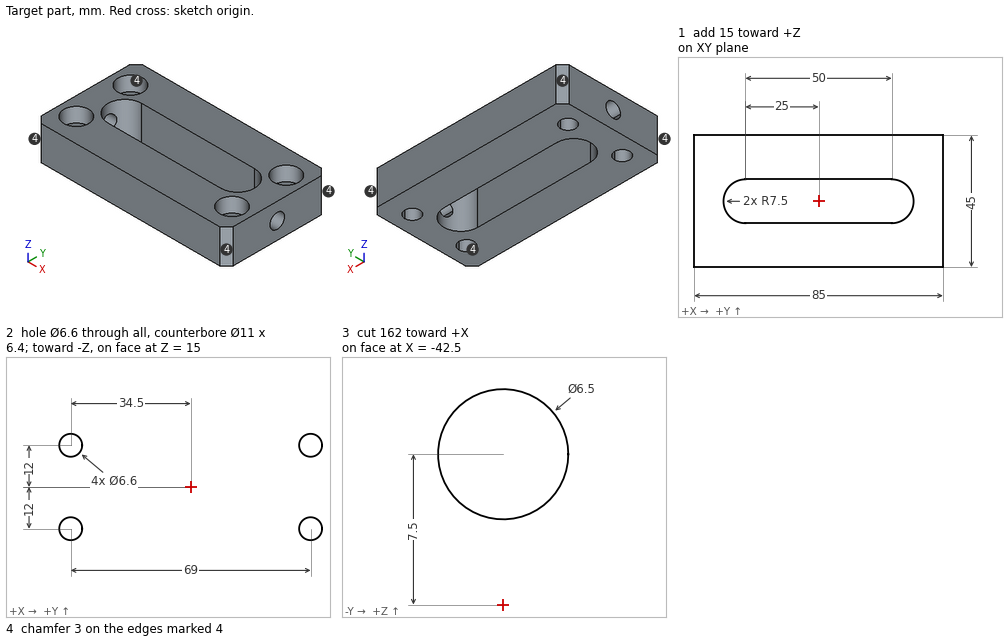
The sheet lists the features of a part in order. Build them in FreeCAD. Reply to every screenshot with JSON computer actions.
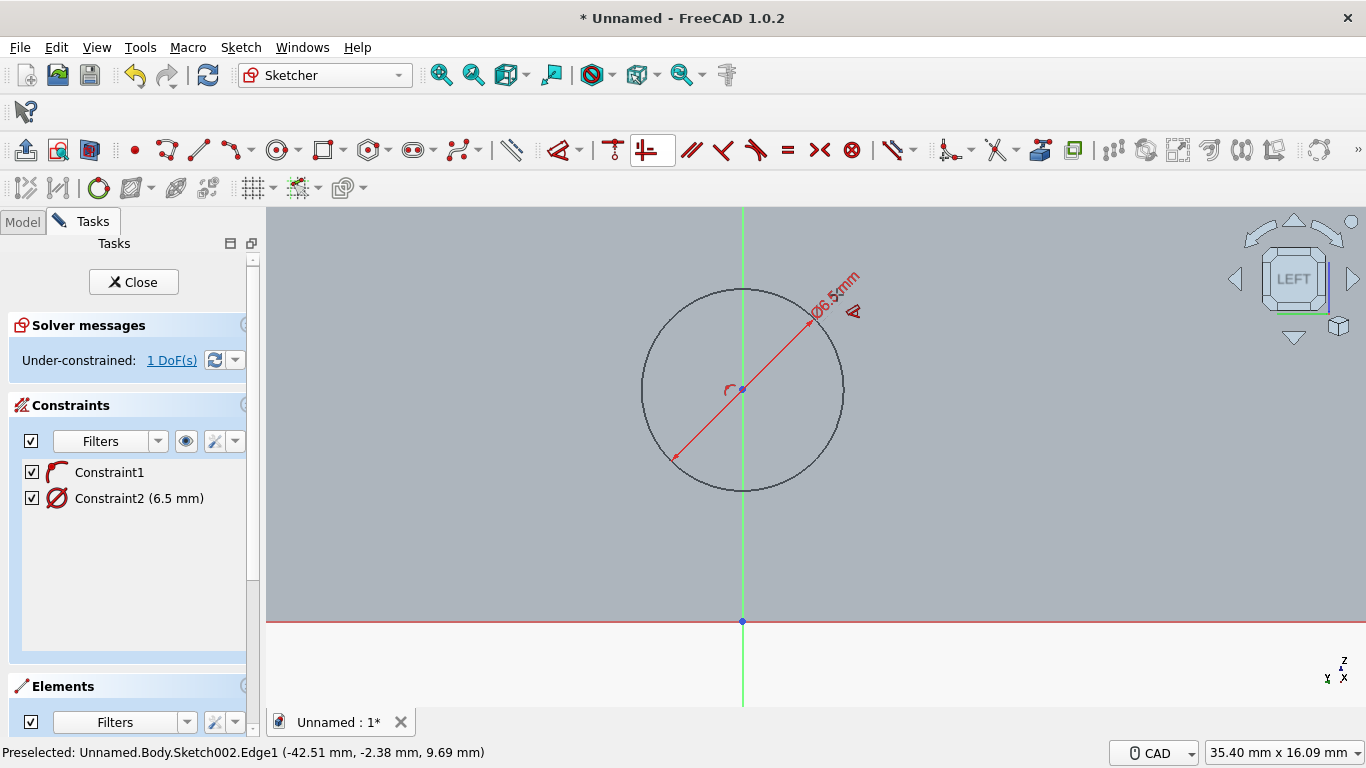
{"action": "left_click", "coordinate": [743, 390]}
{"action": "left_click", "coordinate": [777, 506]}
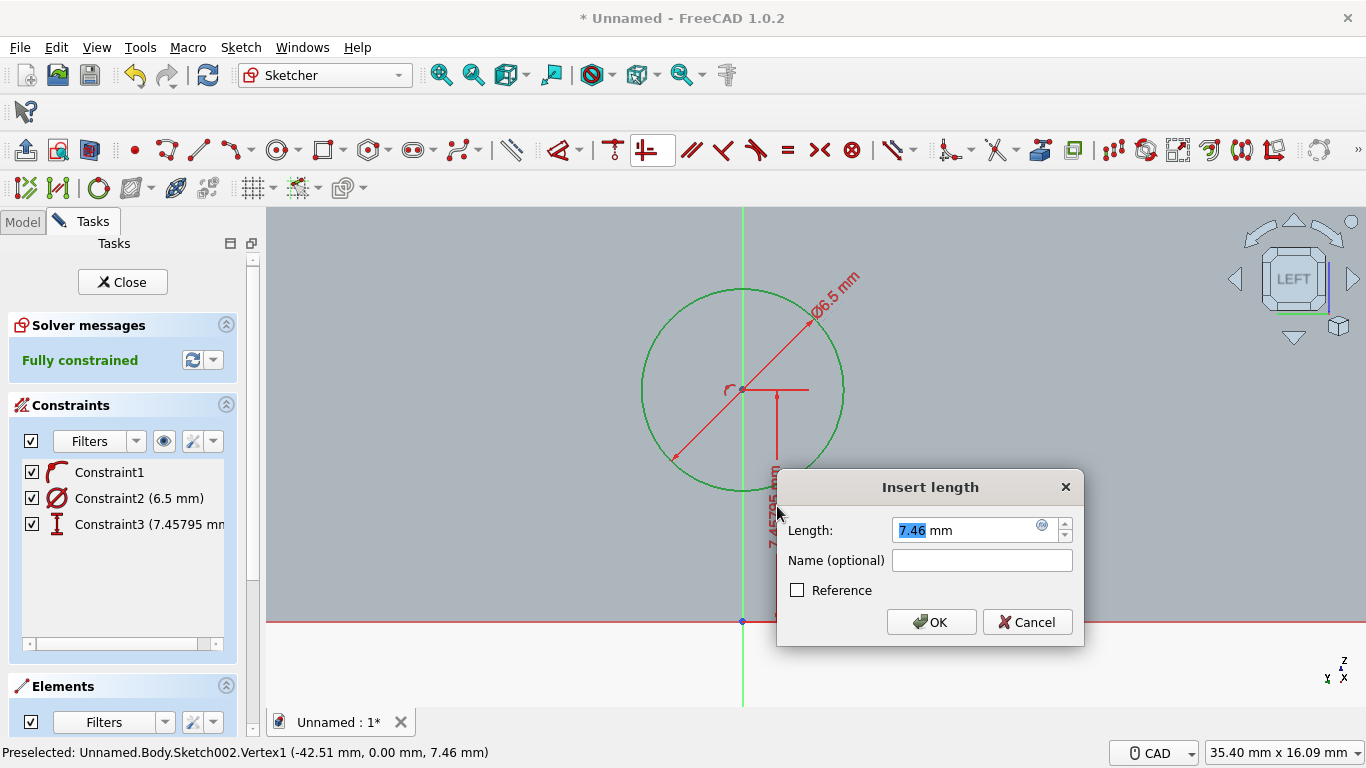
{"action": "type", "text": "7.5"}
{"action": "key", "text": "Return"}
{"action": "key", "text": "Escape"}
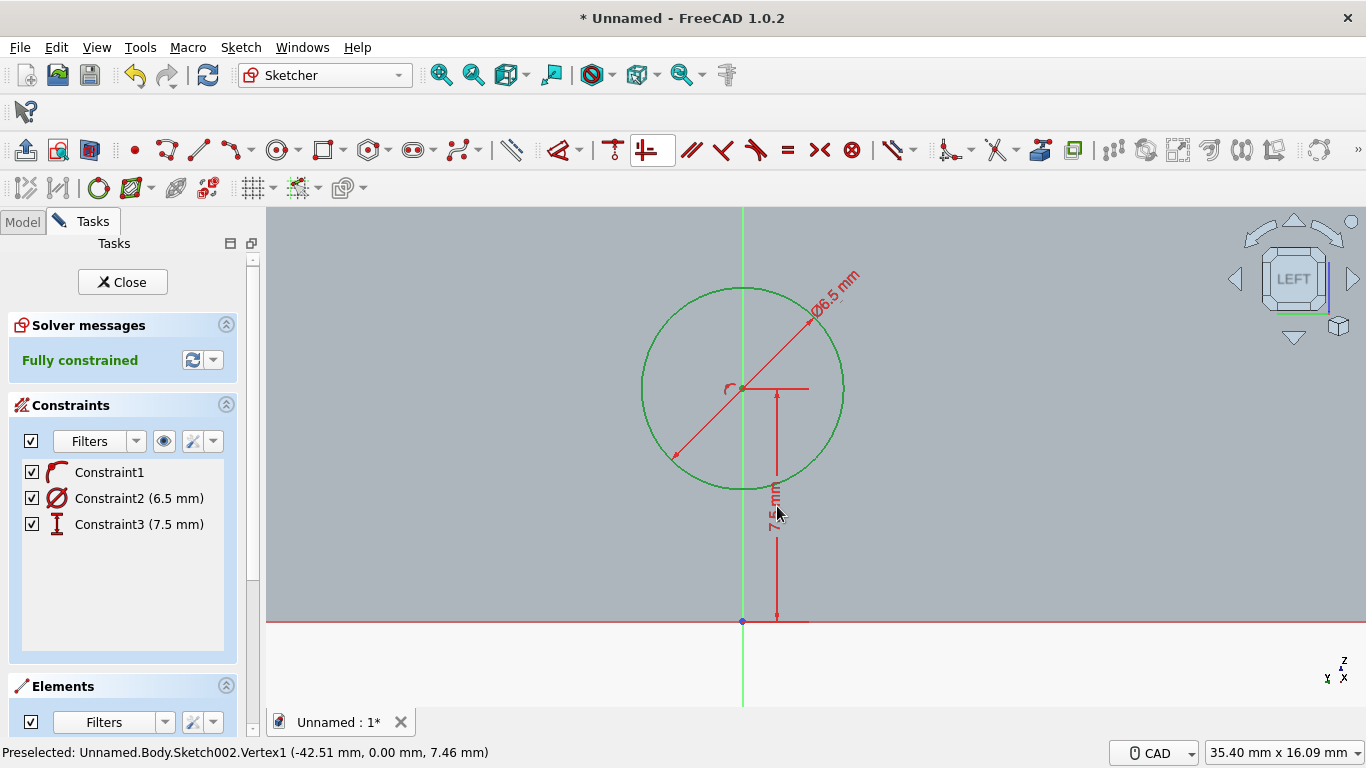
{"action": "left_click", "coordinate": [123, 282]}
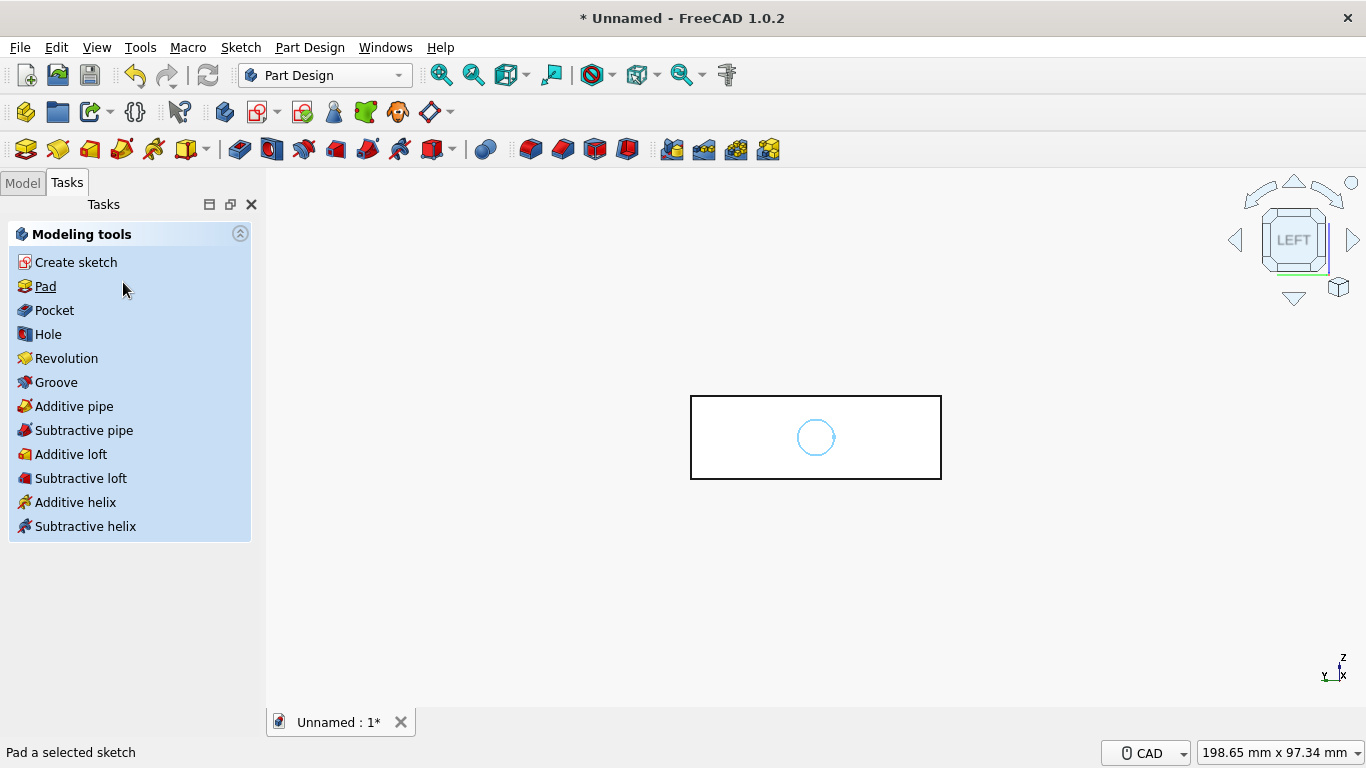
{"action": "left_click", "coordinate": [240, 150]}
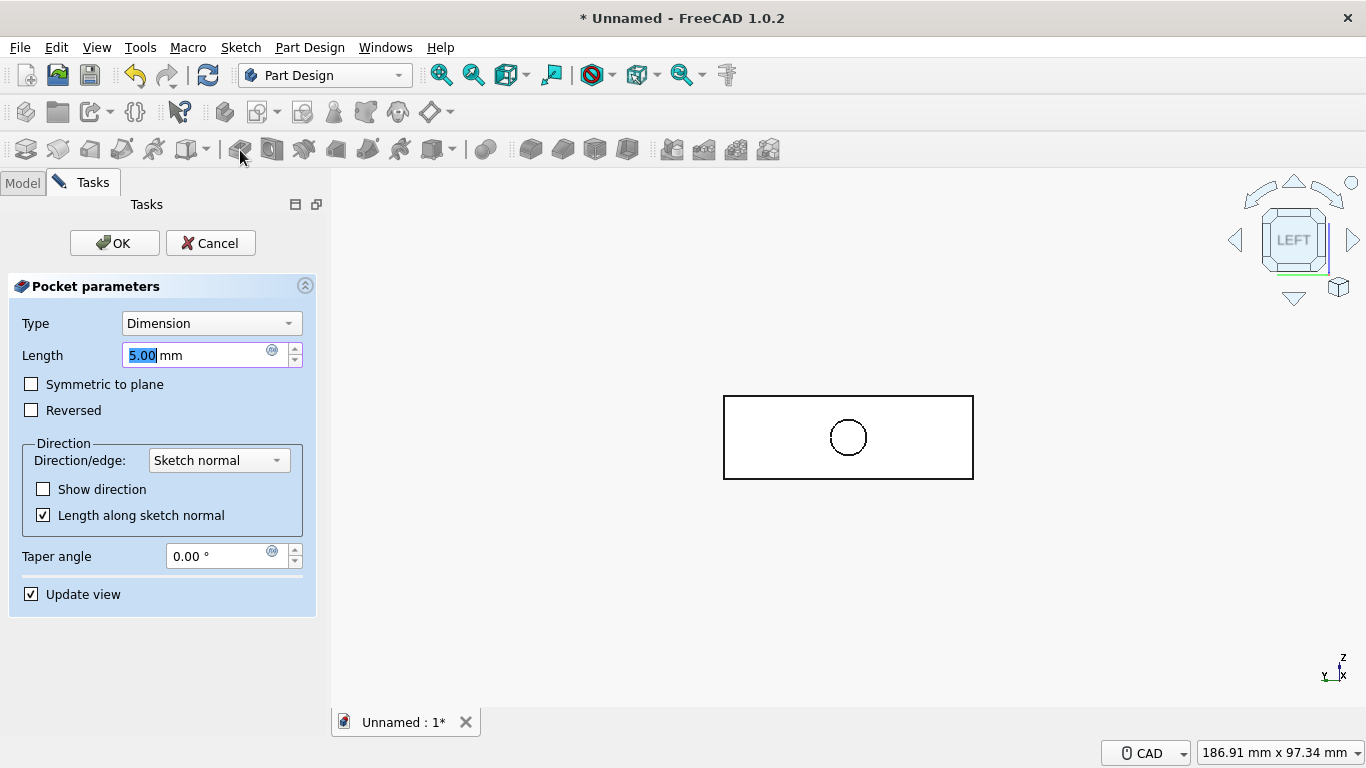
{"action": "type", "text": "162"}
{"action": "key", "text": "Tab"}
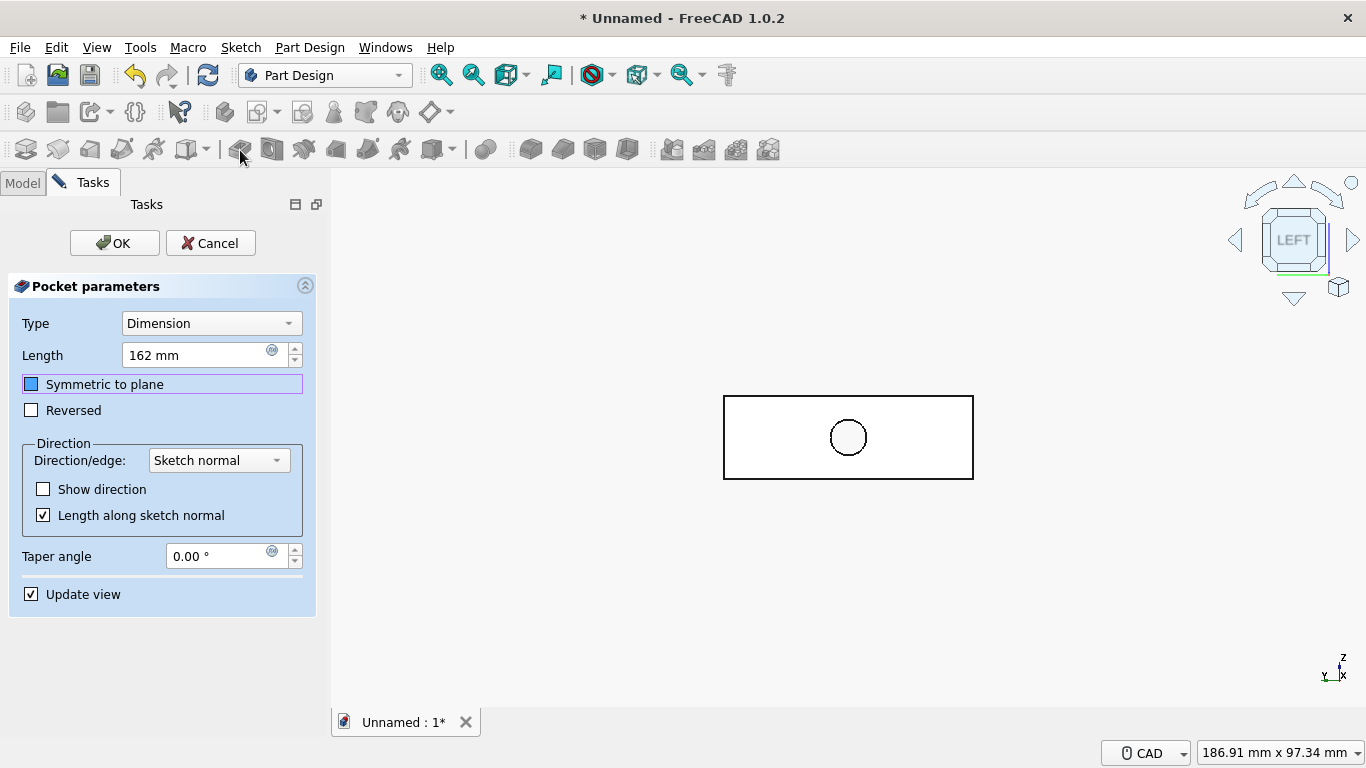
{"action": "left_click", "coordinate": [115, 243]}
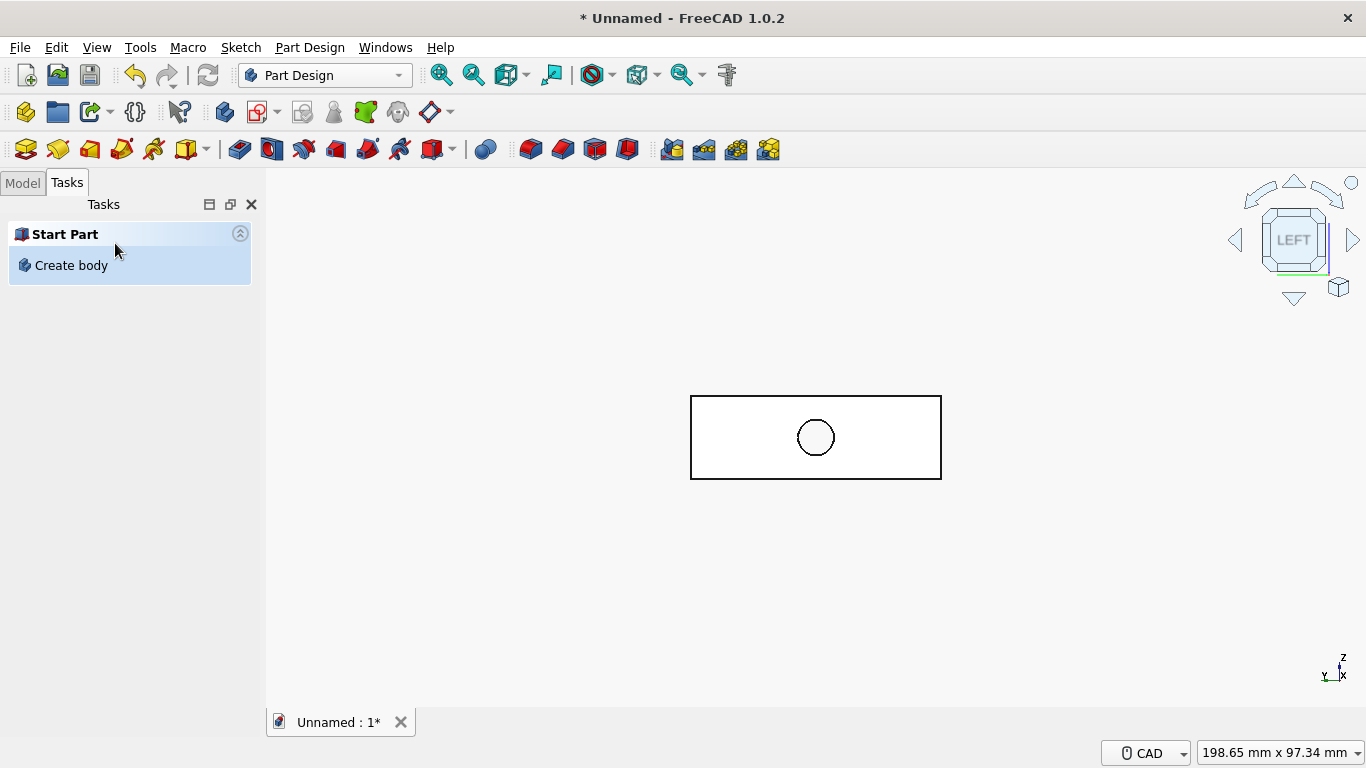
{"action": "left_click", "coordinate": [442, 76]}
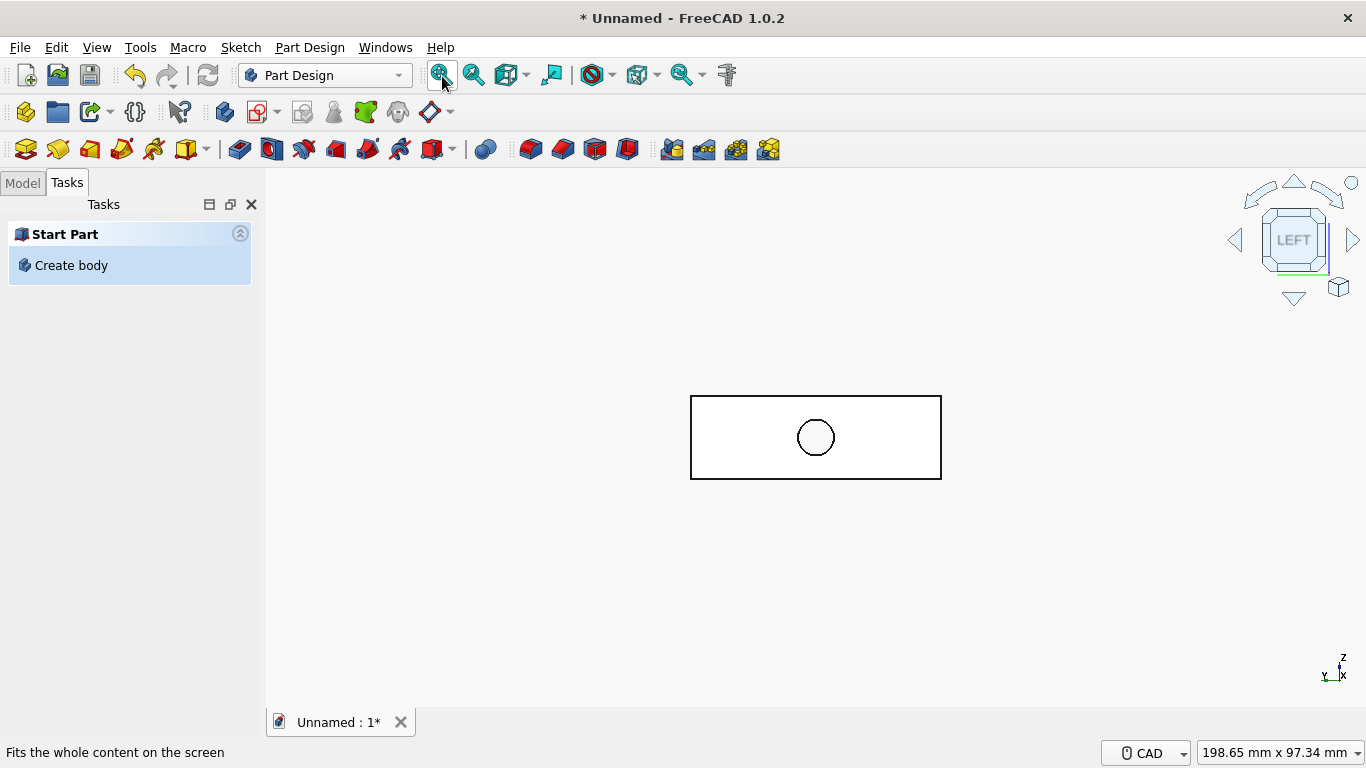
{"action": "left_click", "coordinate": [941, 436]}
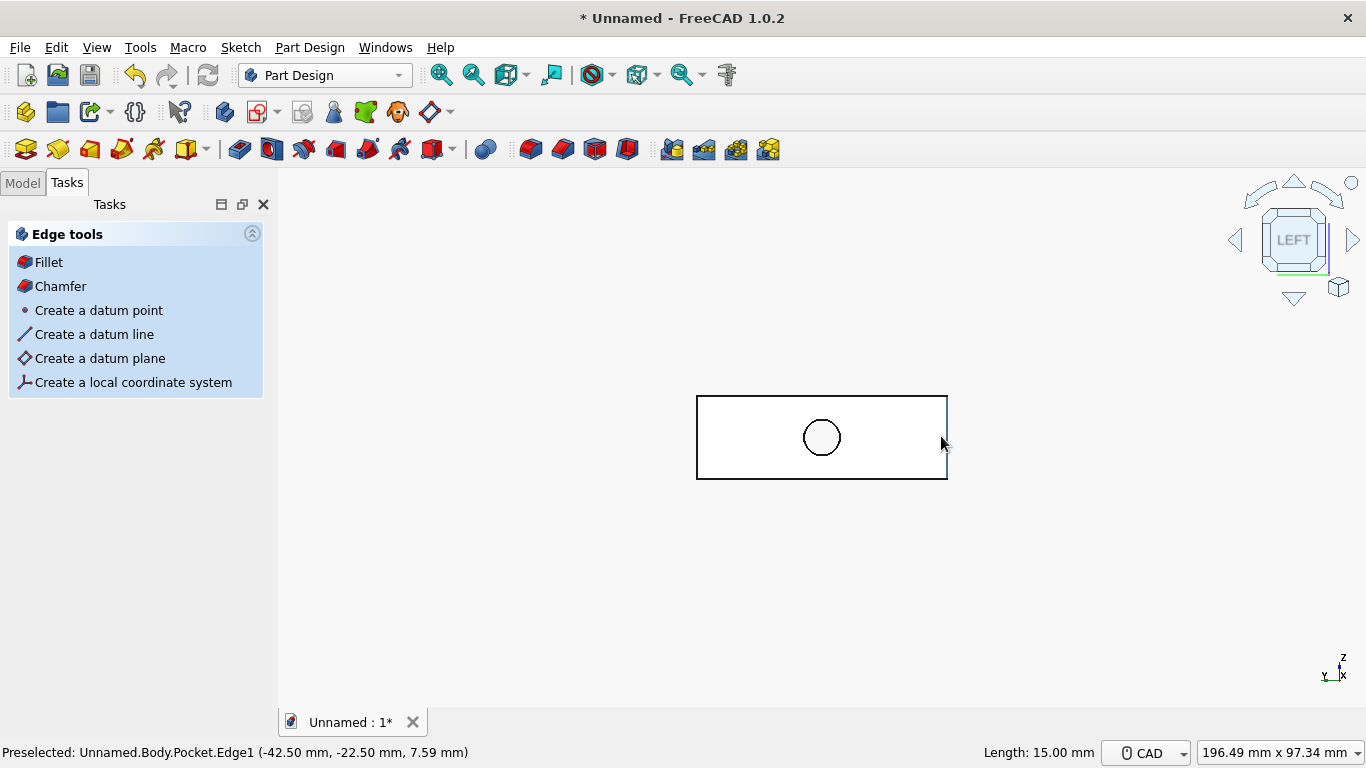
{"action": "left_click", "coordinate": [697, 436], "text": "ctrl"}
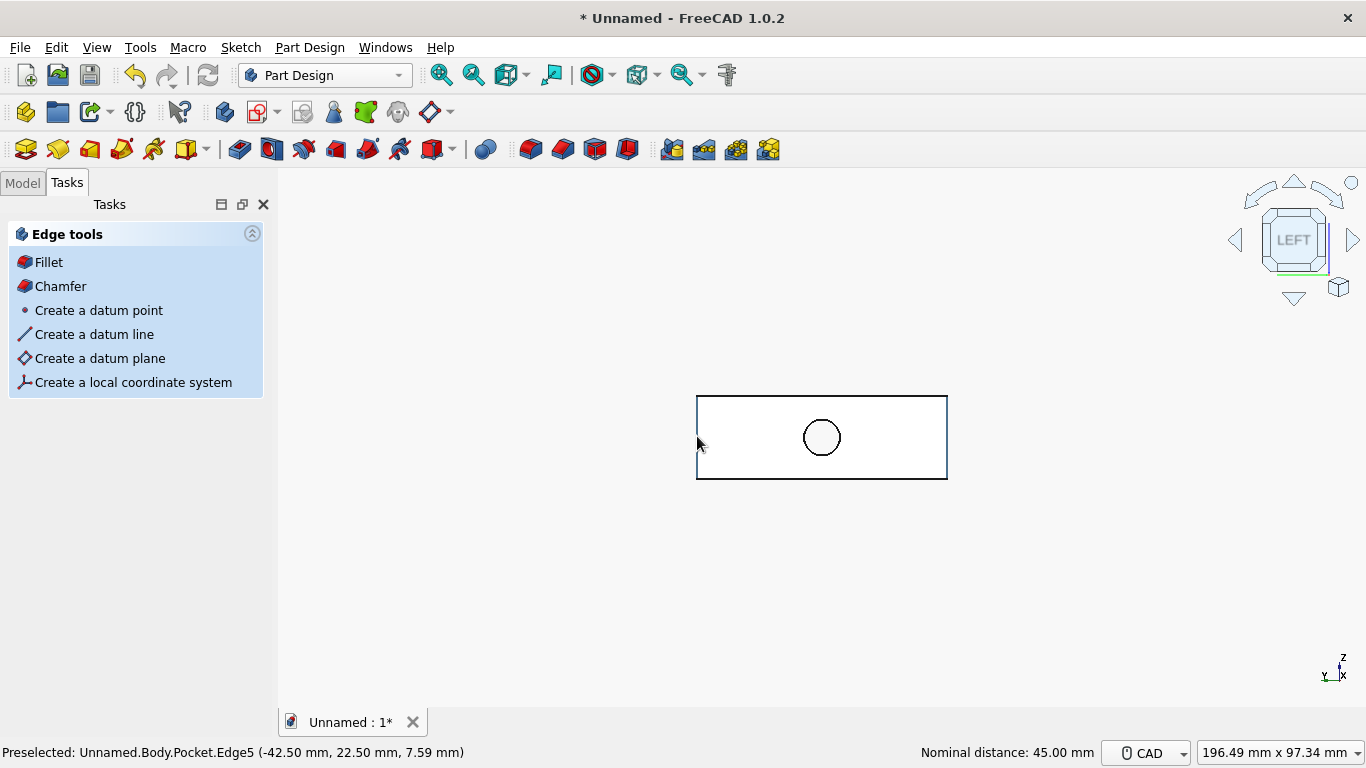
{"action": "key", "text": "0"}